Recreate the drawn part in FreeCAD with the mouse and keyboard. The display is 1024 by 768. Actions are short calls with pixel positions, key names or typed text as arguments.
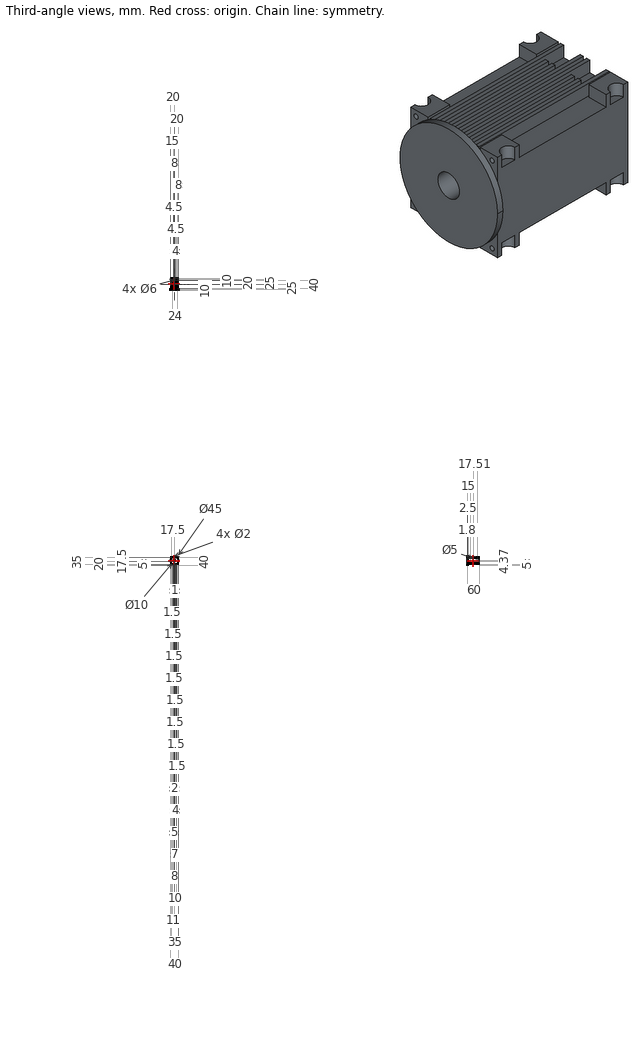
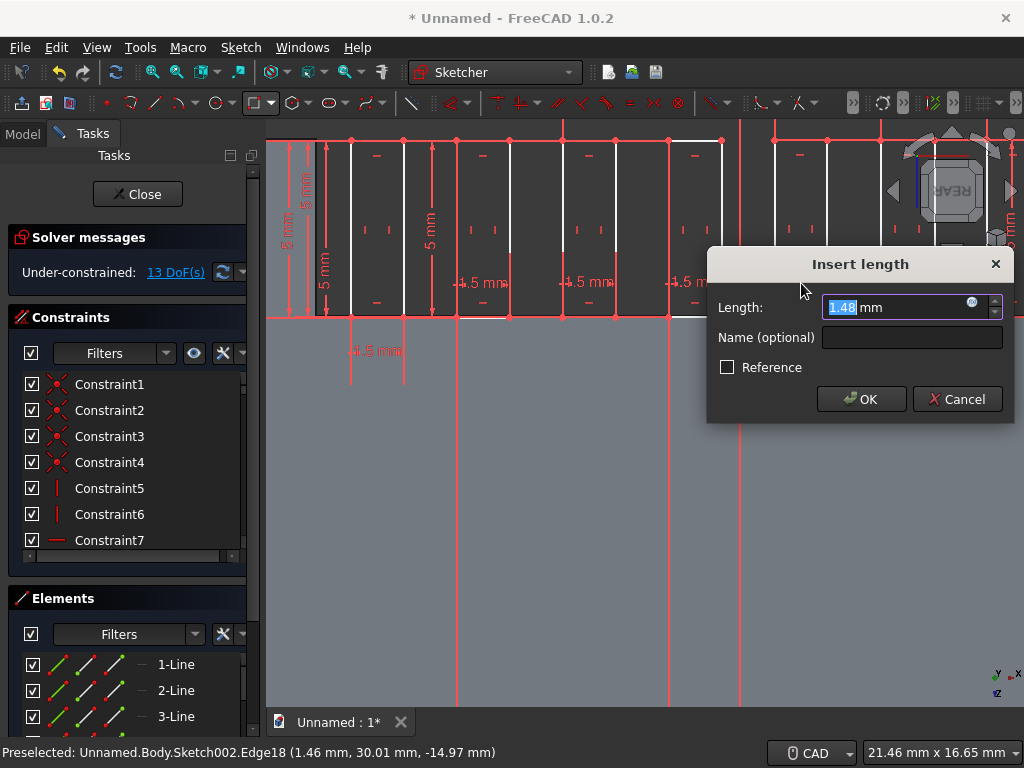
text(1.5)
key(Return)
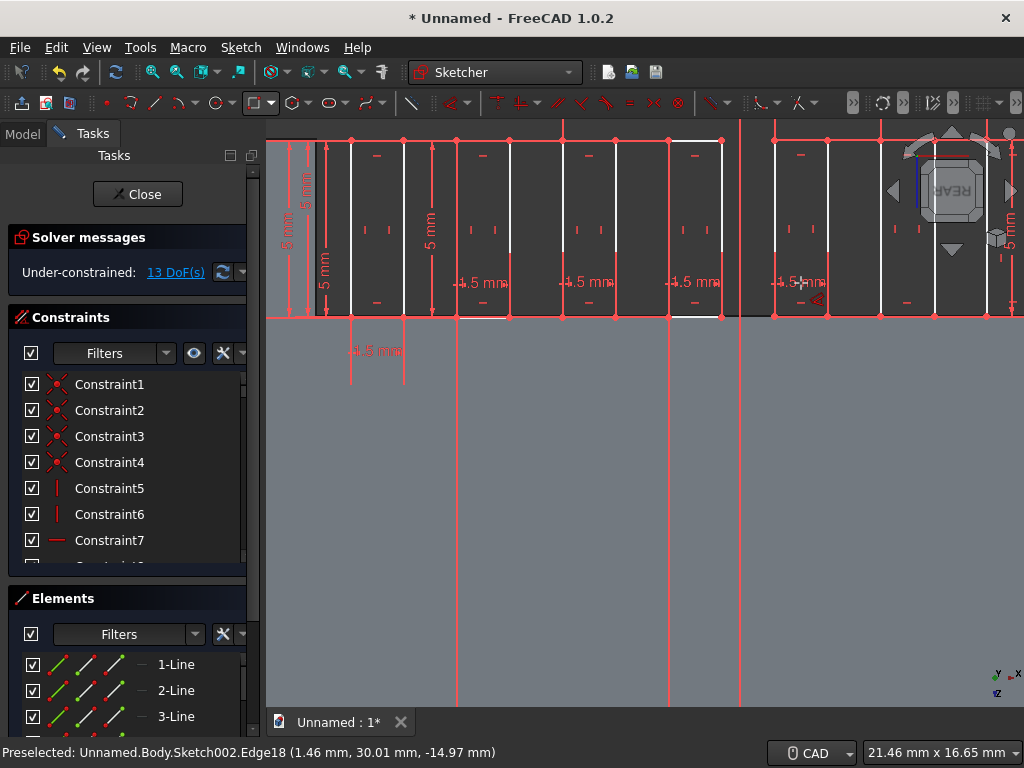
scroll(367, 317, down, 3)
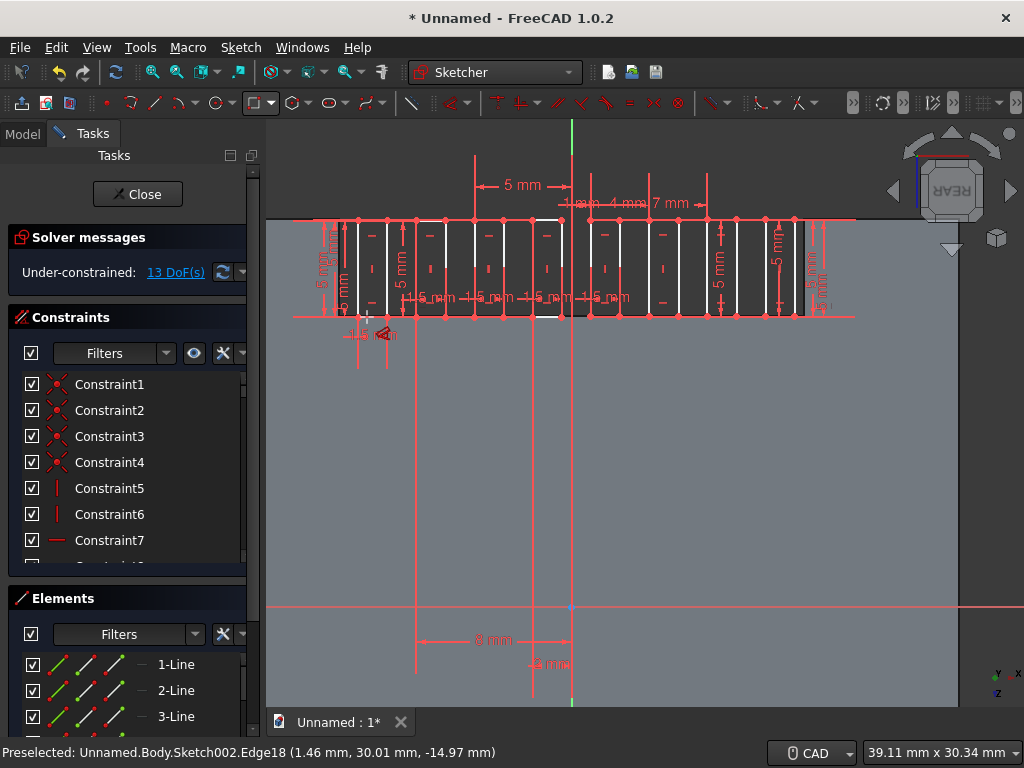
scroll(658, 317, up, 3)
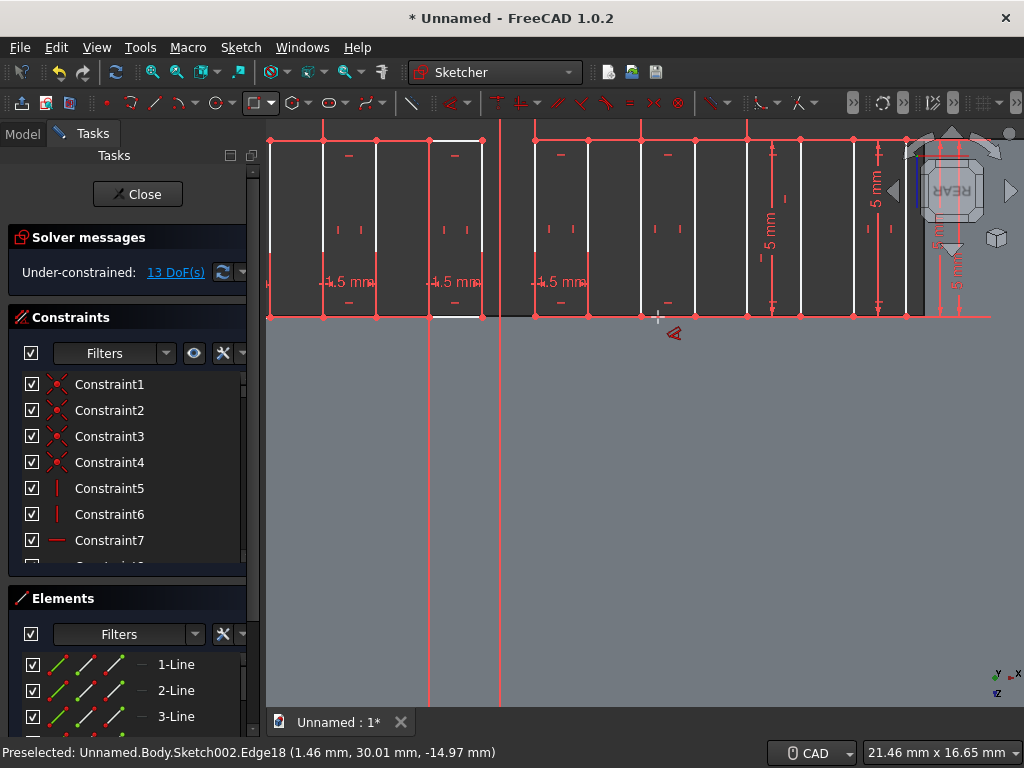
click(657, 317)
click(668, 283)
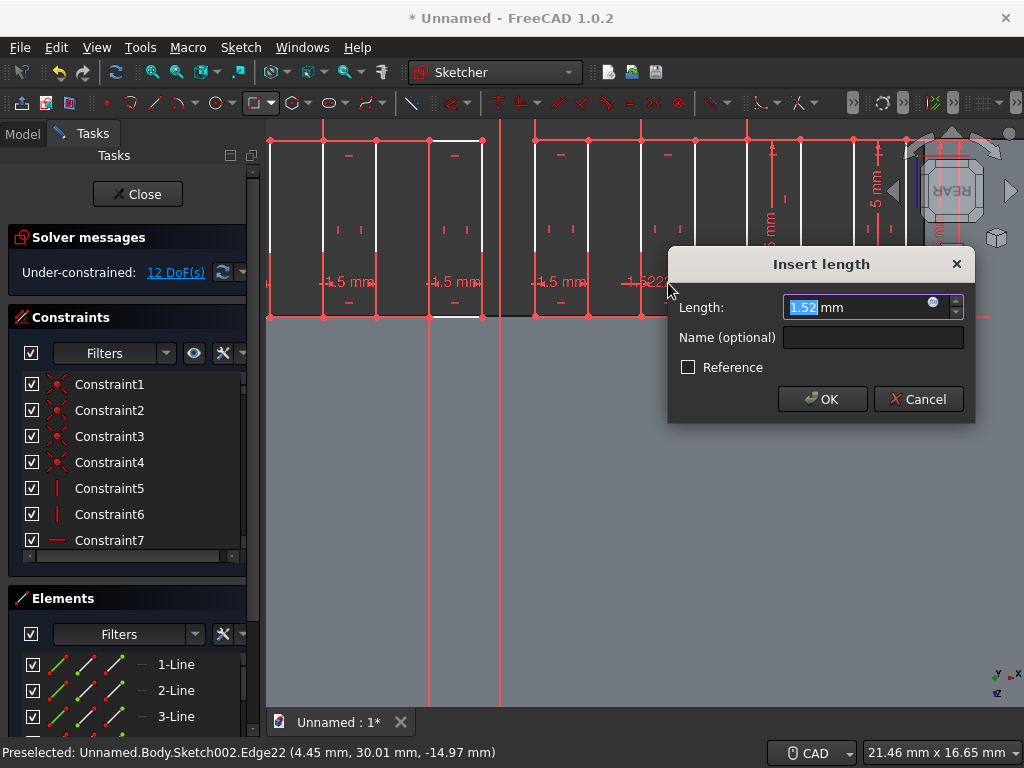
text(1.5)
key(Return)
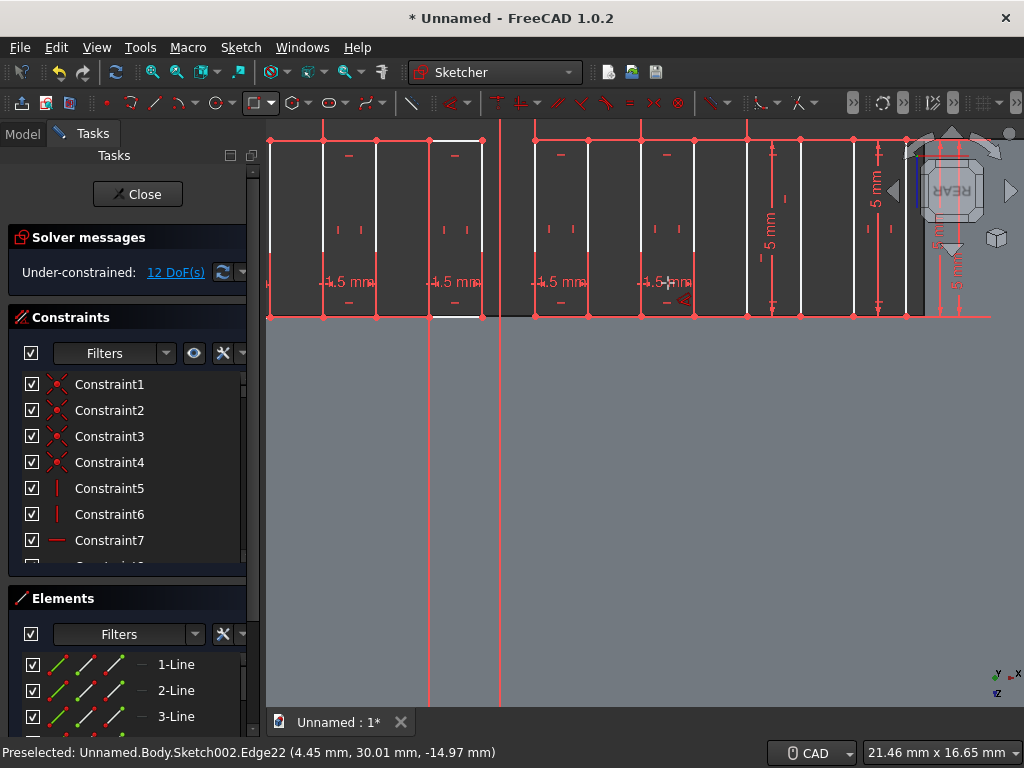
click(763, 317)
click(774, 283)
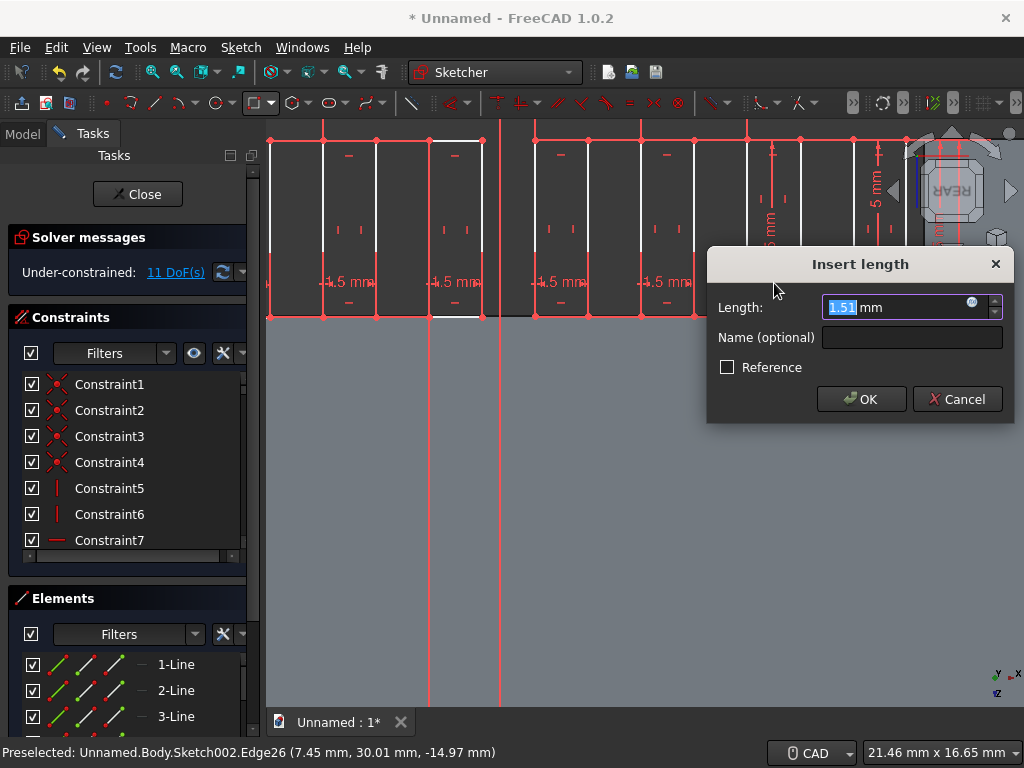
text(1.5)
key(Return)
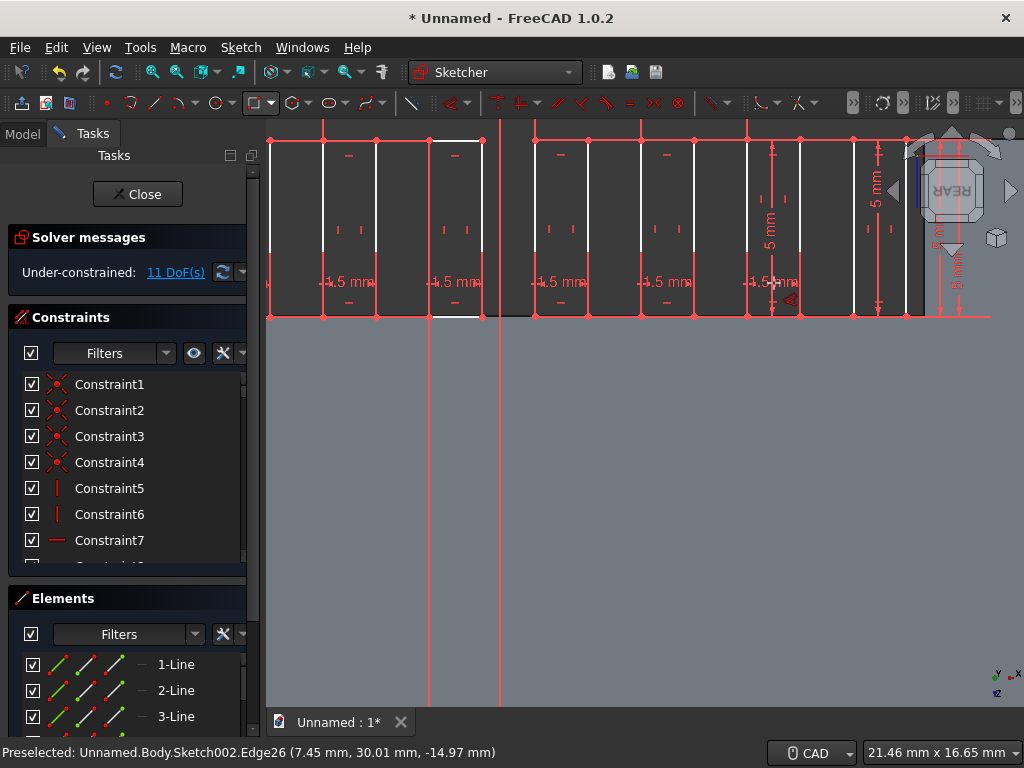
scroll(659, 317, down, 3)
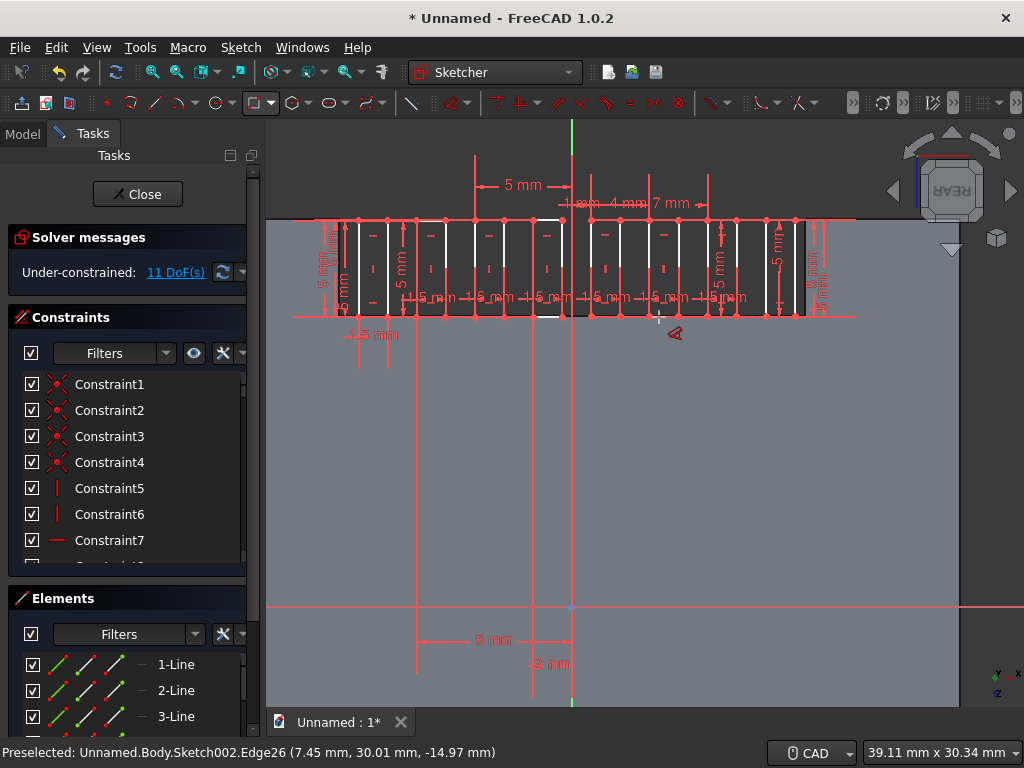
scroll(775, 317, up, 3)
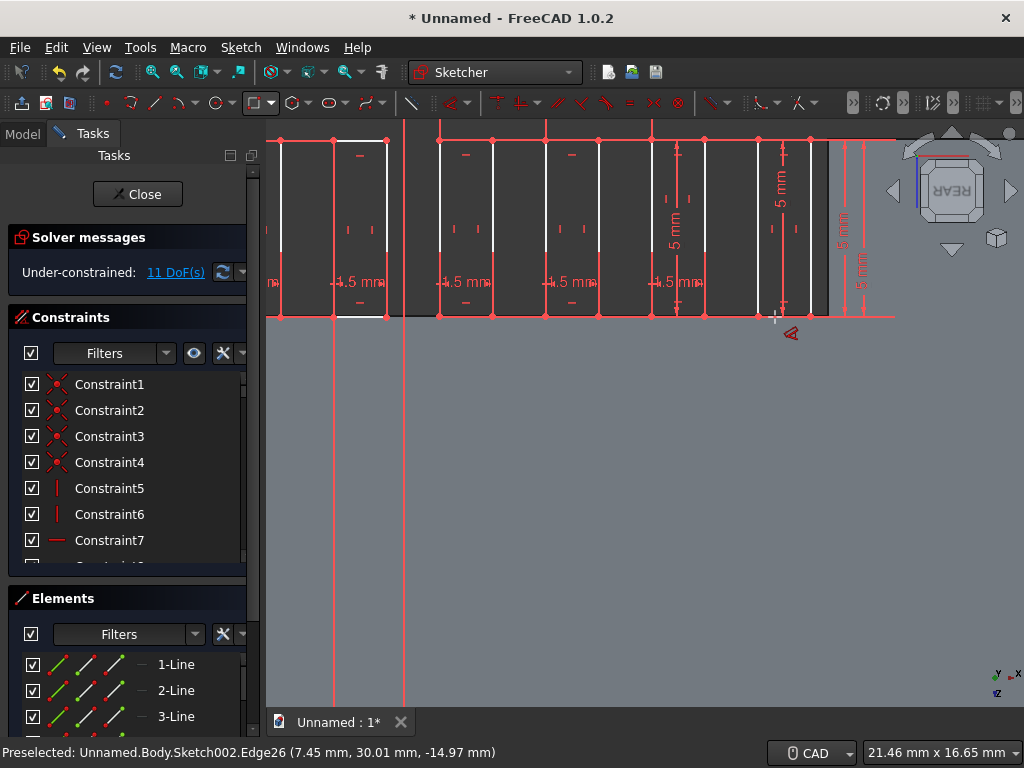
click(774, 317)
click(784, 283)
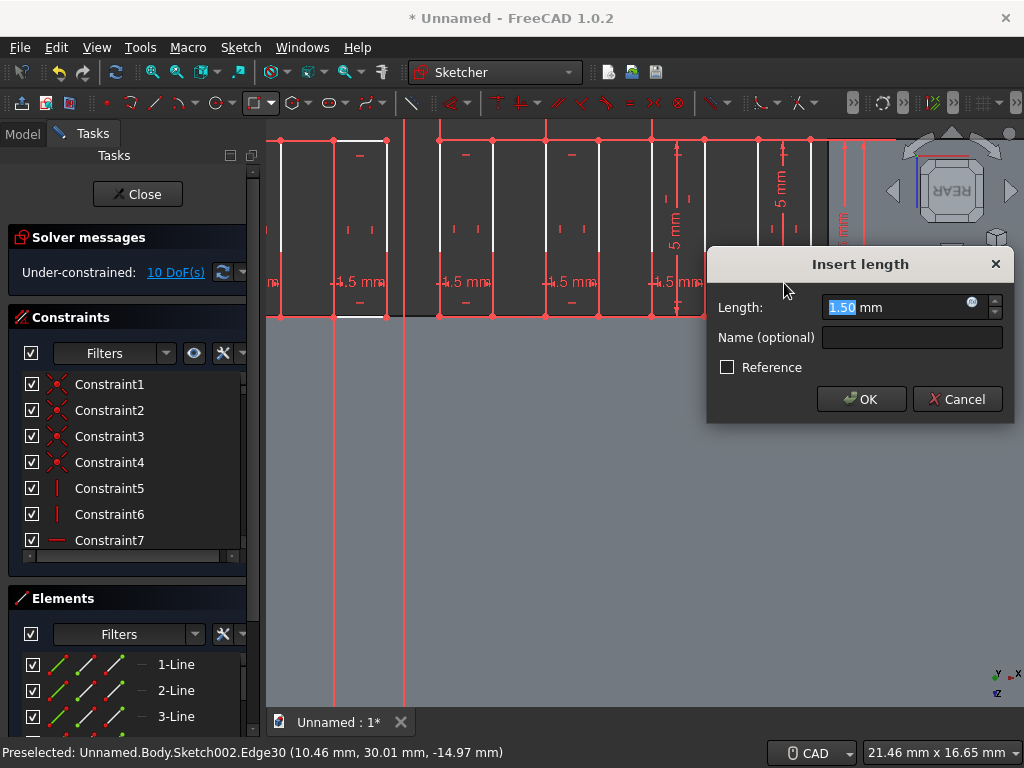
text(1.5)
key(Return)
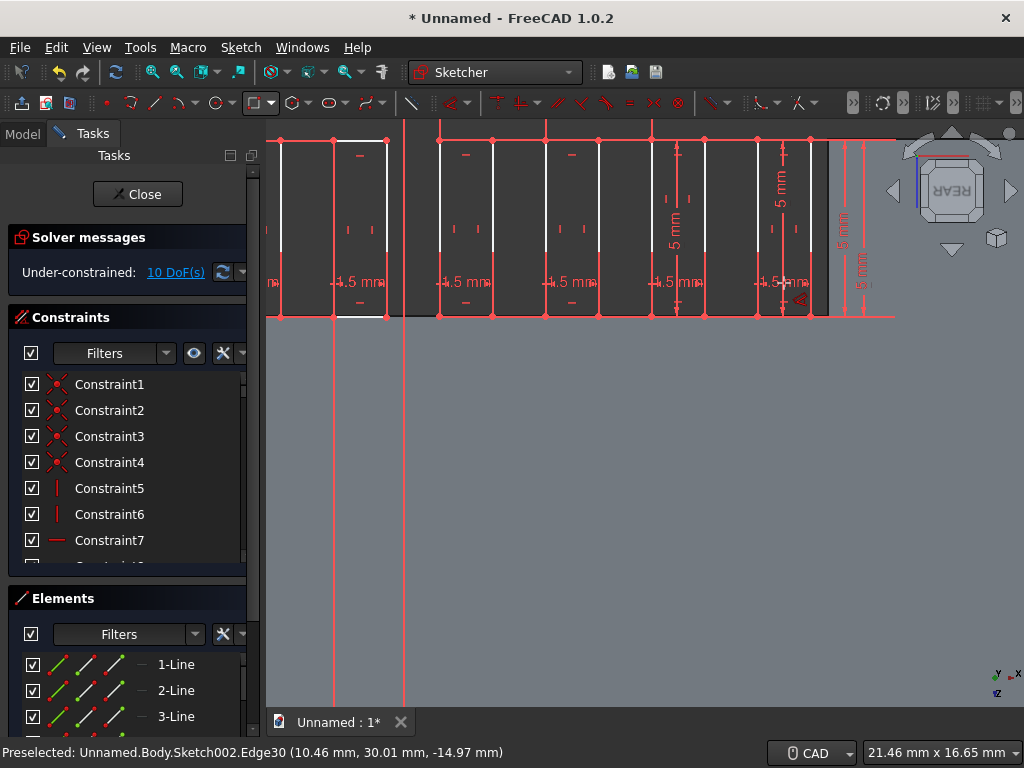
scroll(775, 317, down, 3)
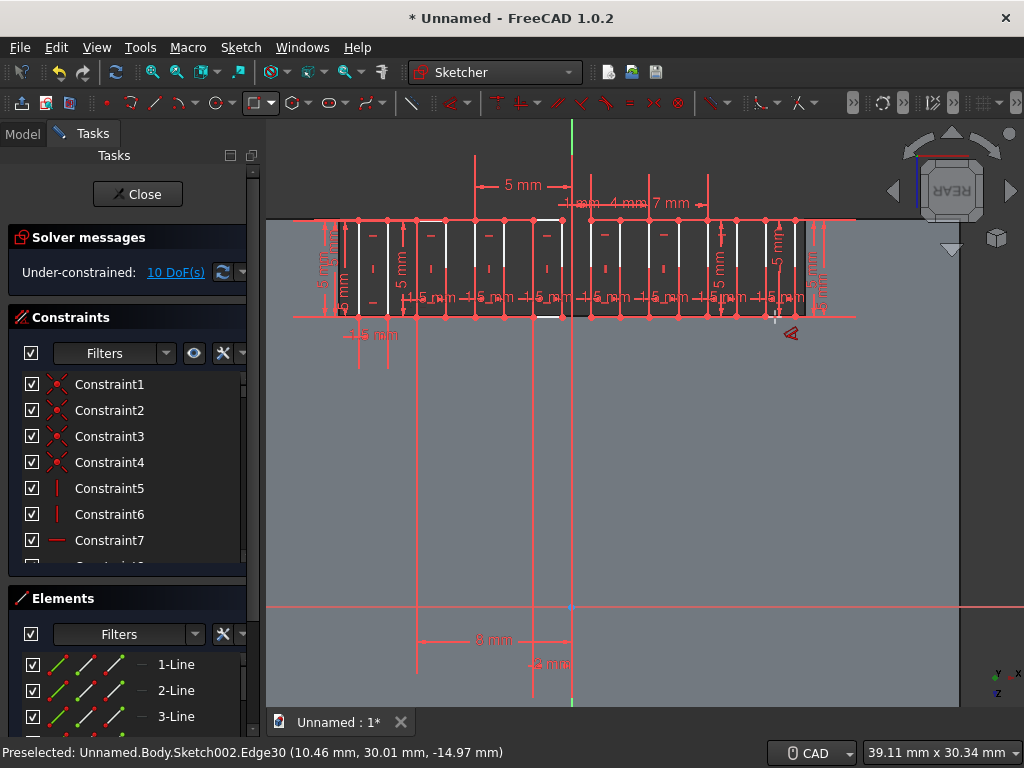
click(359, 221)
click(416, 641)